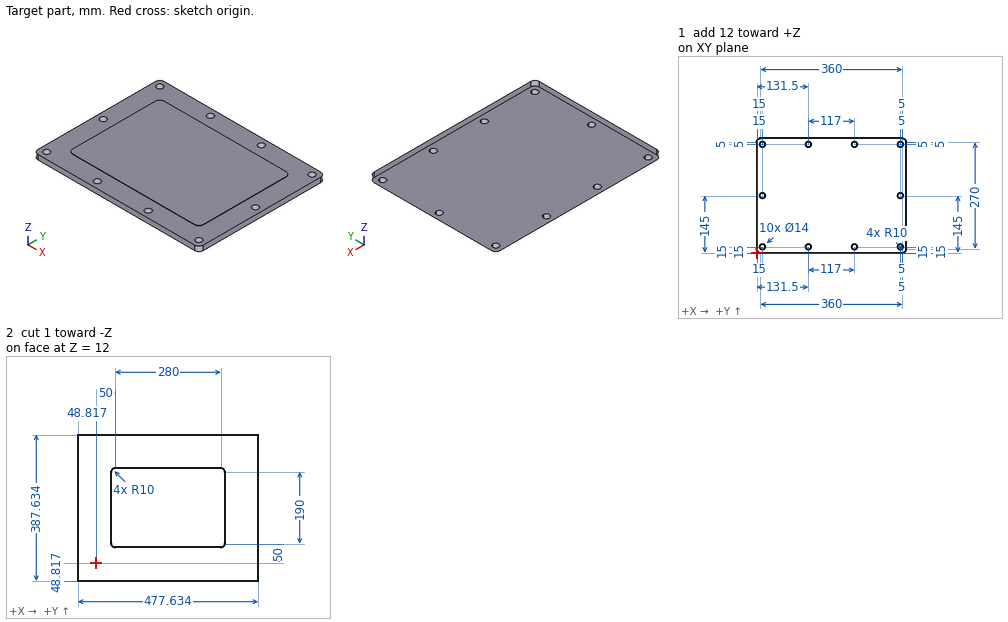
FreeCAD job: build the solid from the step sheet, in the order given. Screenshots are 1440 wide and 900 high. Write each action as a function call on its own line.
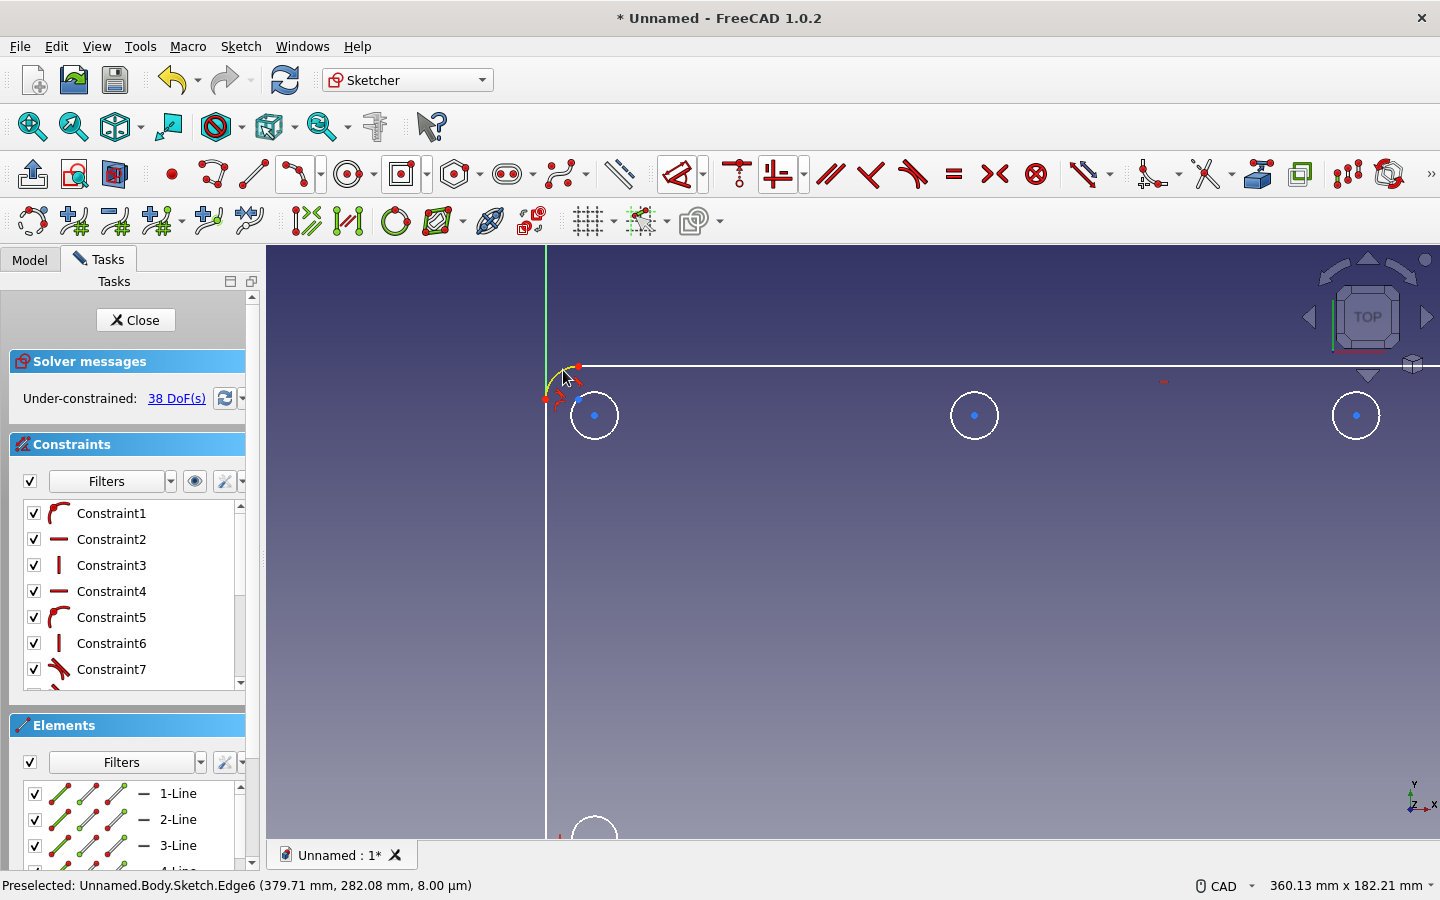
click(564, 370)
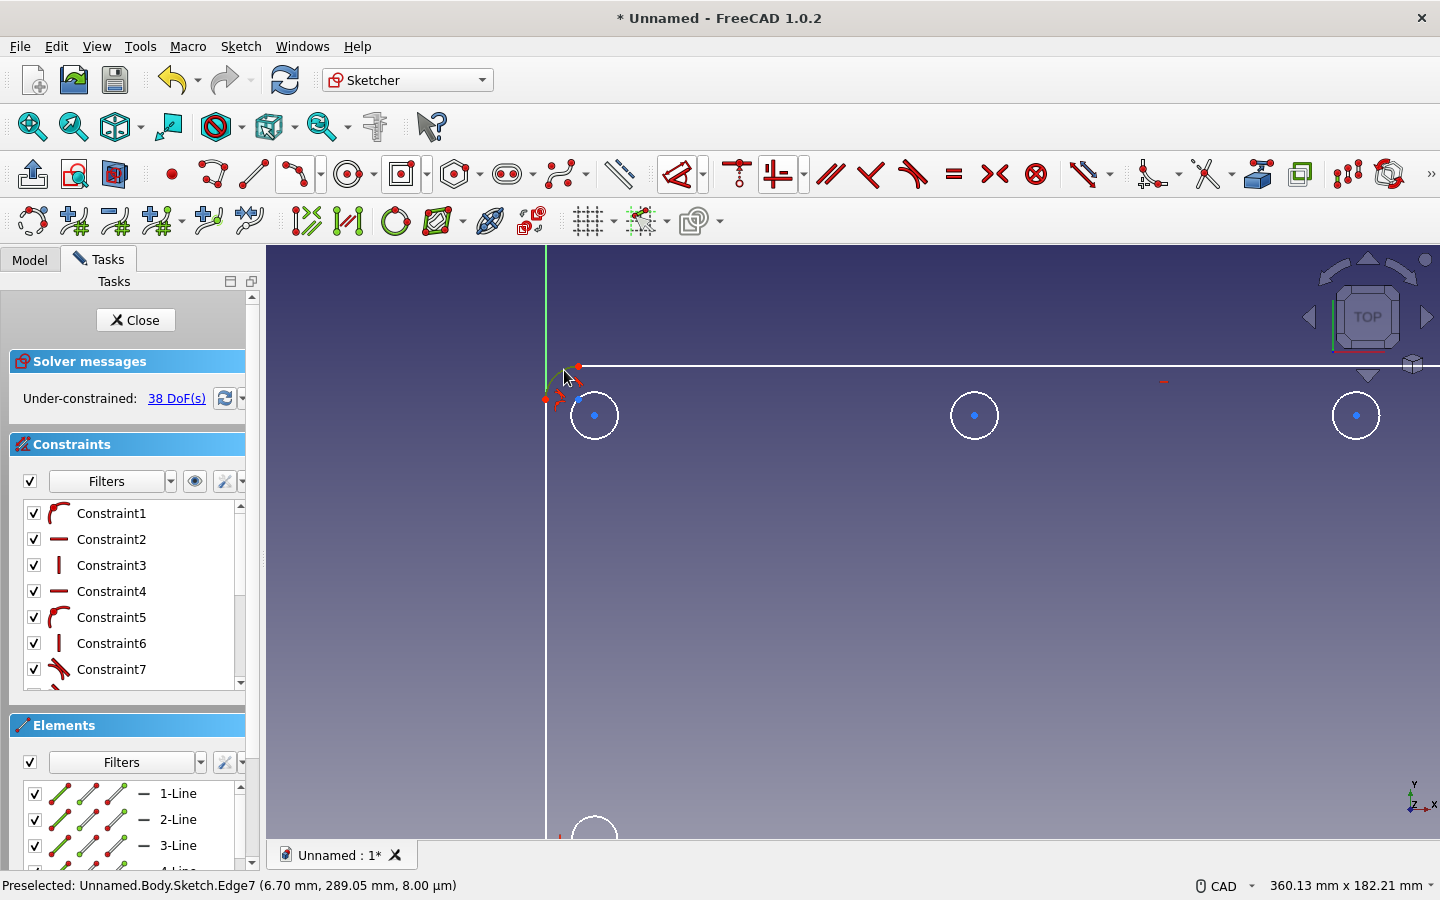
scroll(563, 370, down, 5)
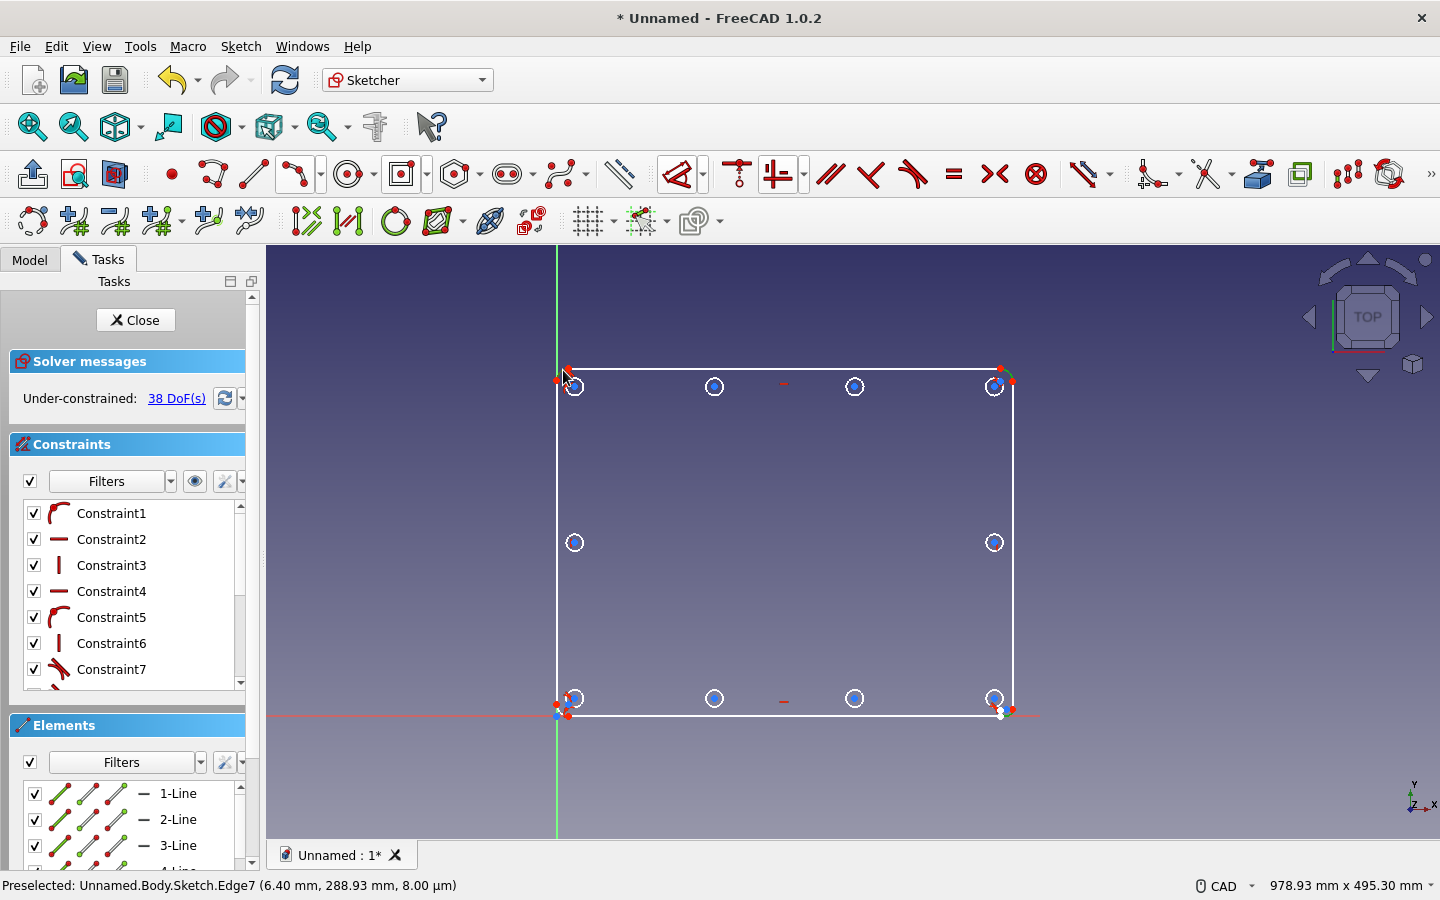
scroll(558, 710, up, 5)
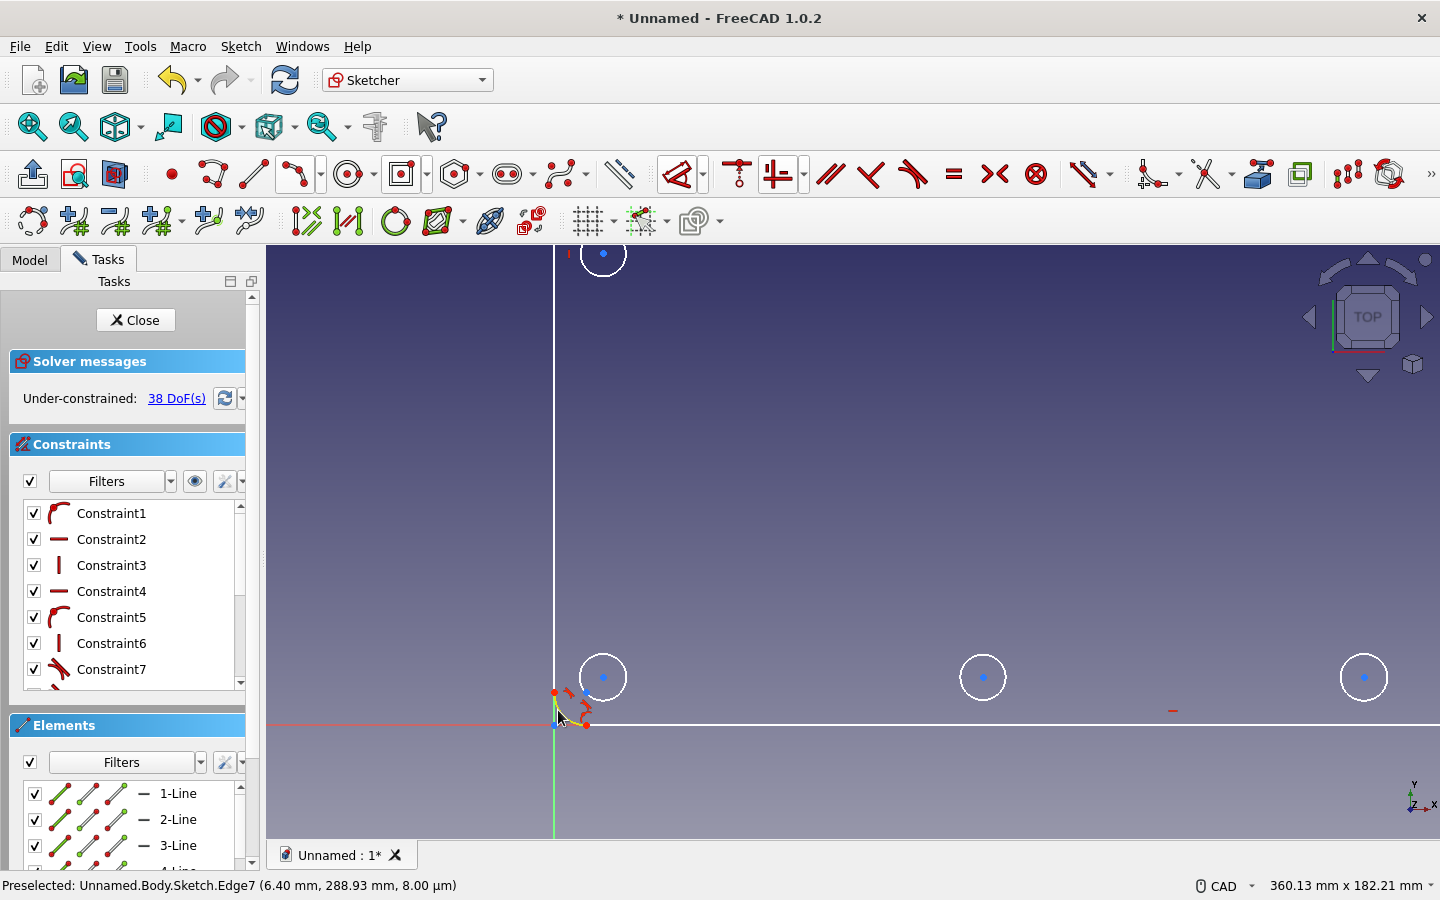
click(558, 708)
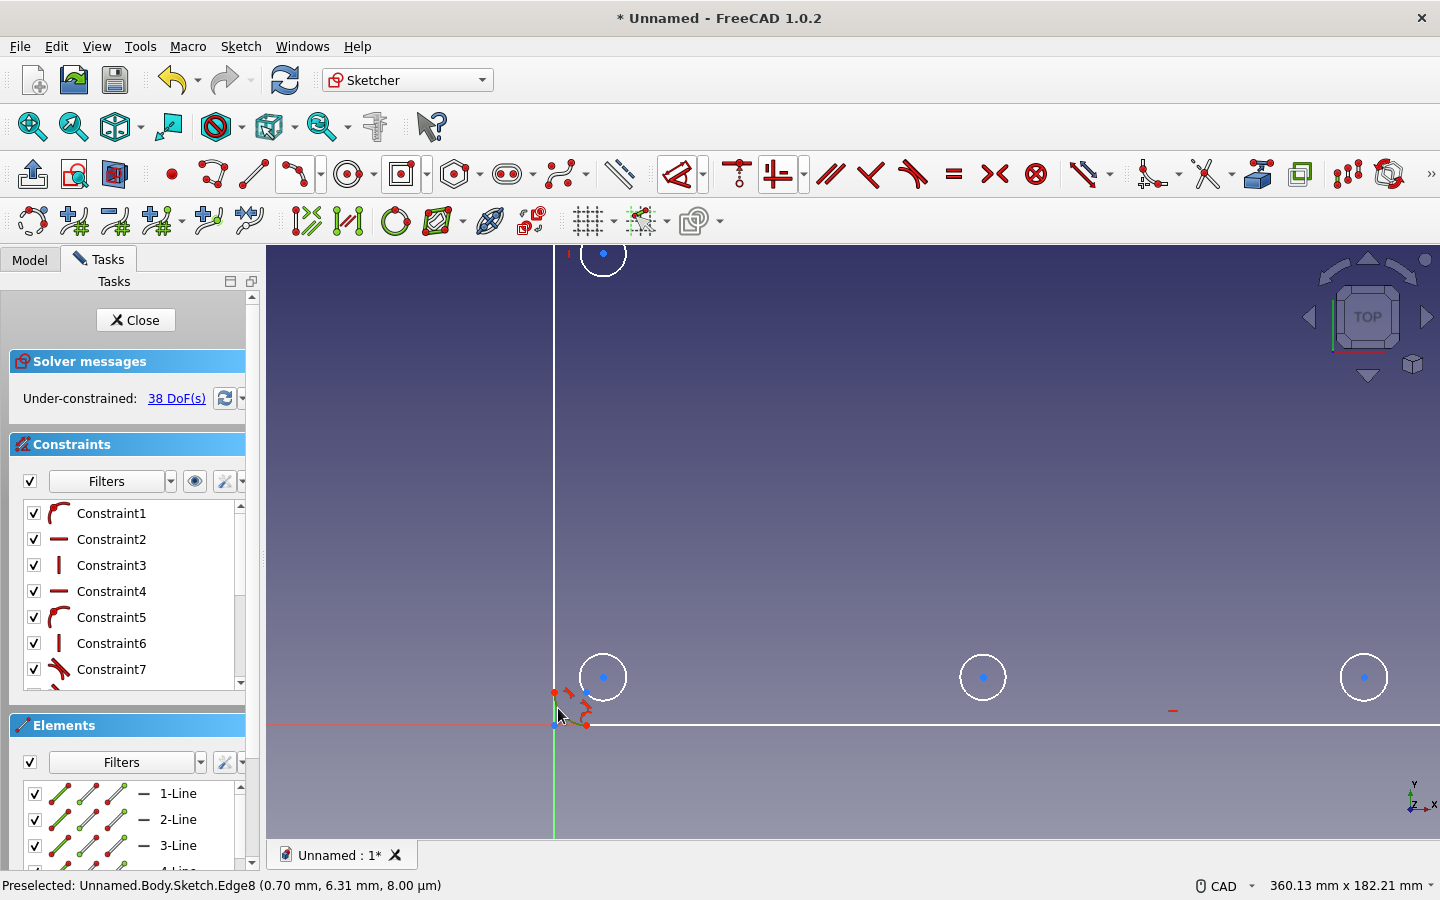
click(954, 174)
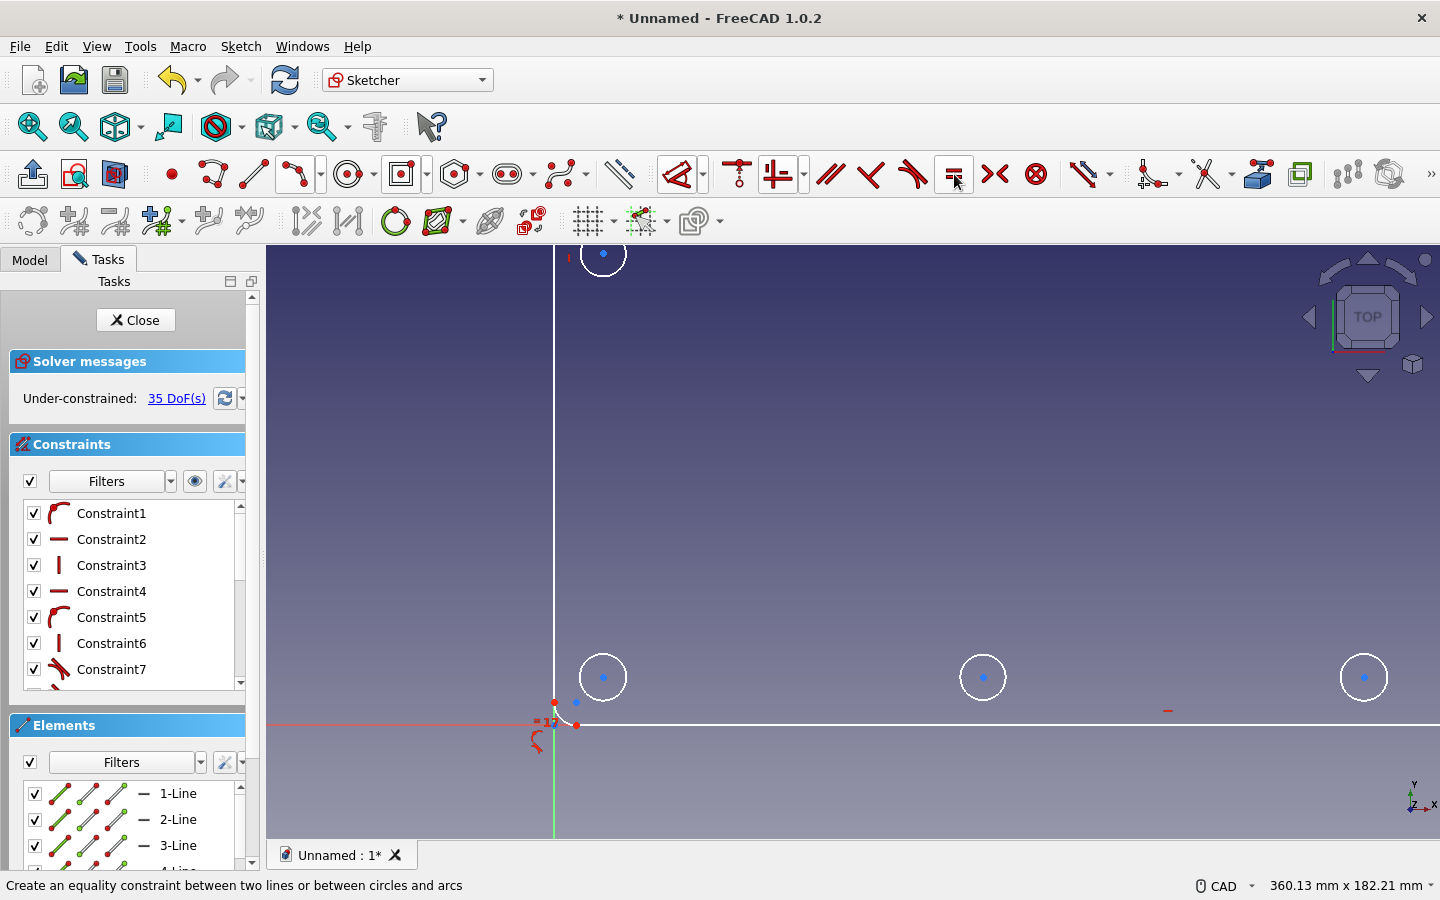
click(619, 661)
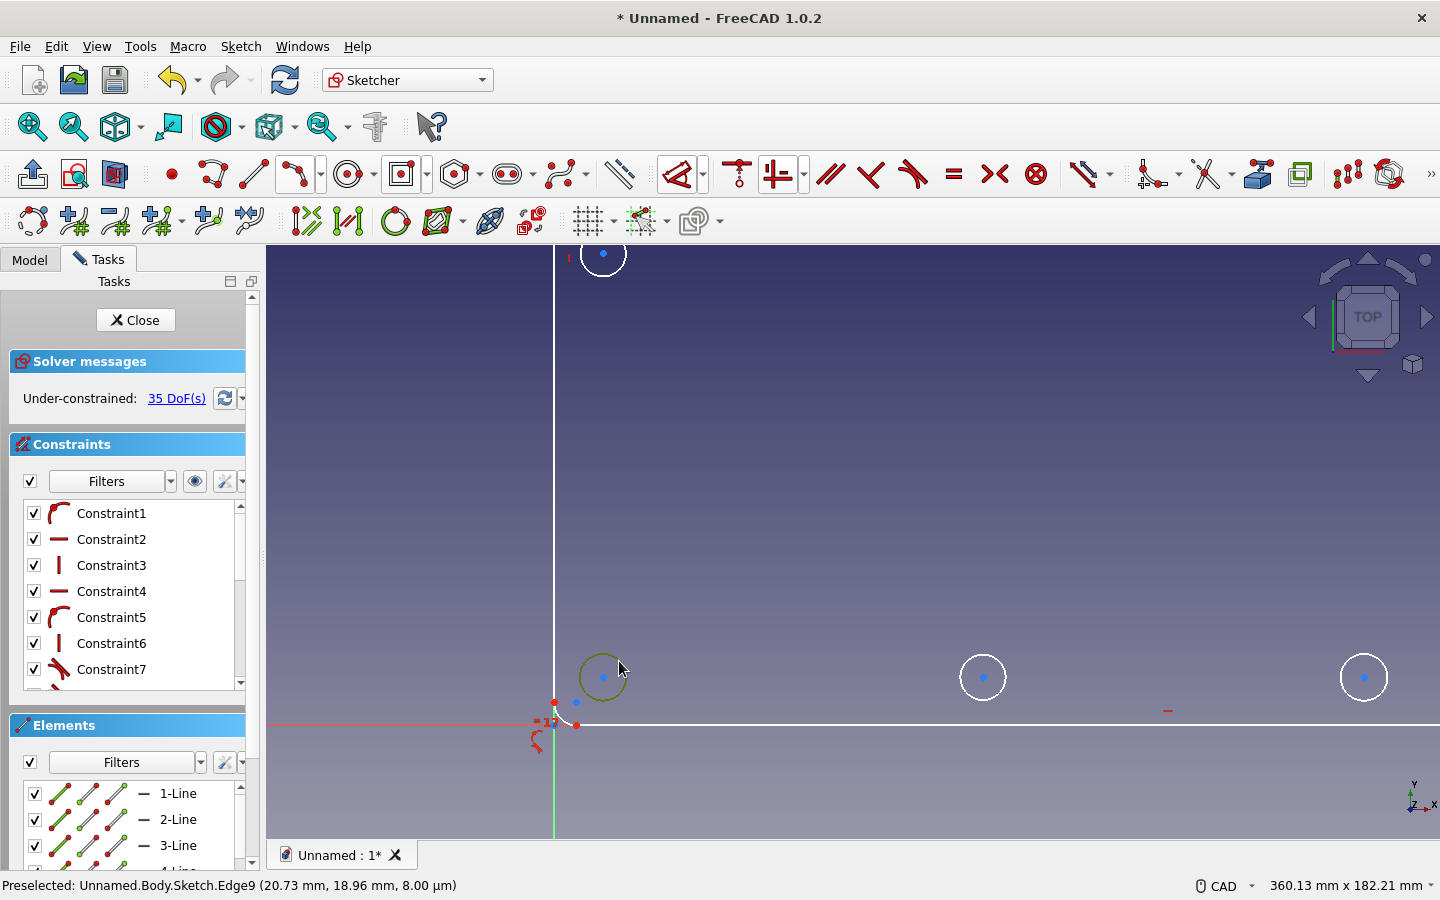
click(999, 661)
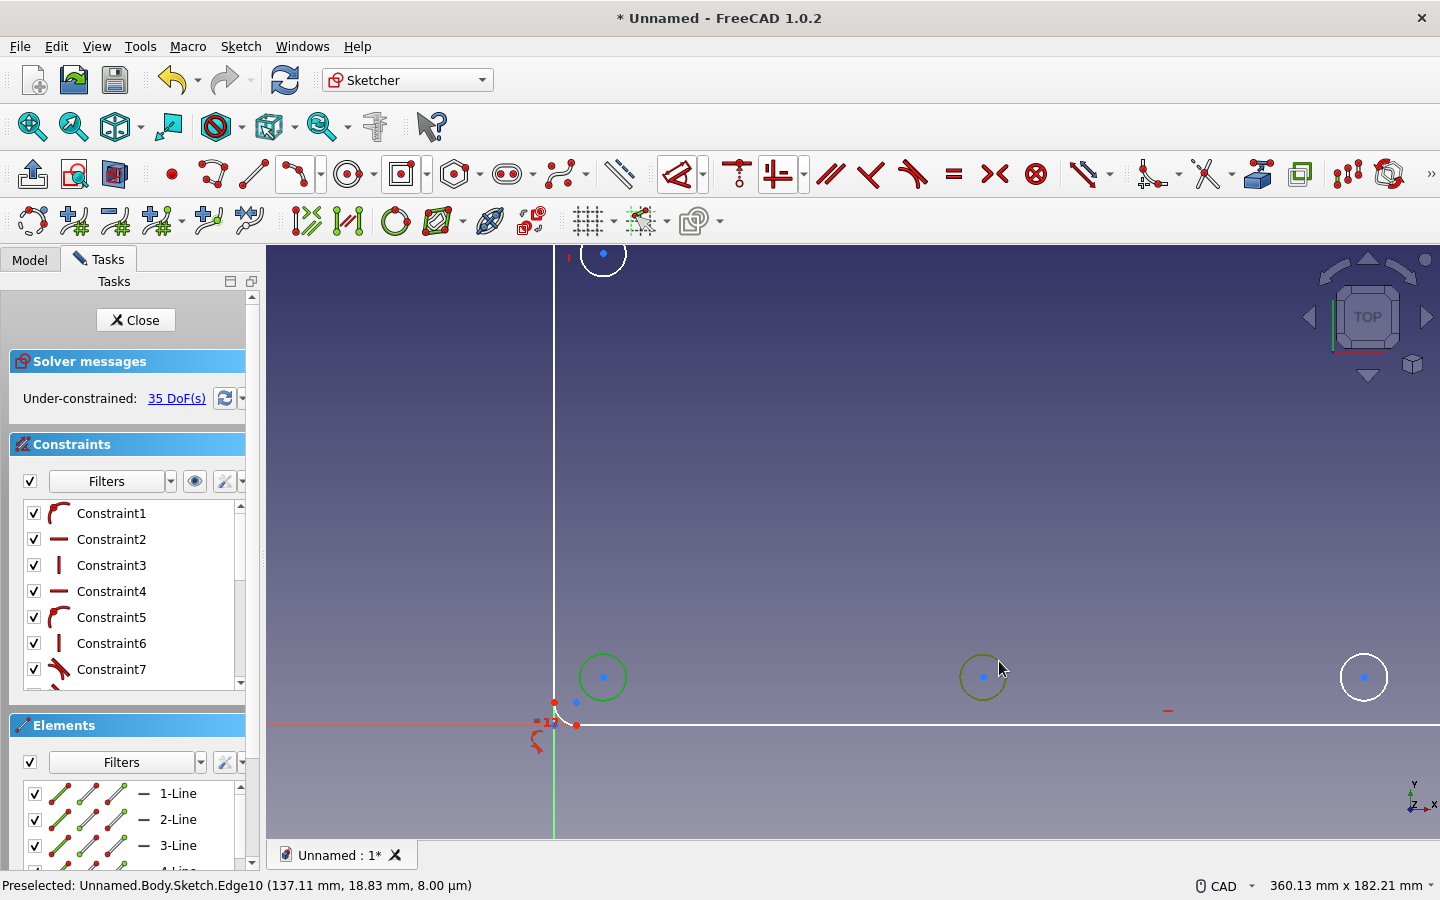
scroll(558, 710, down, 5)